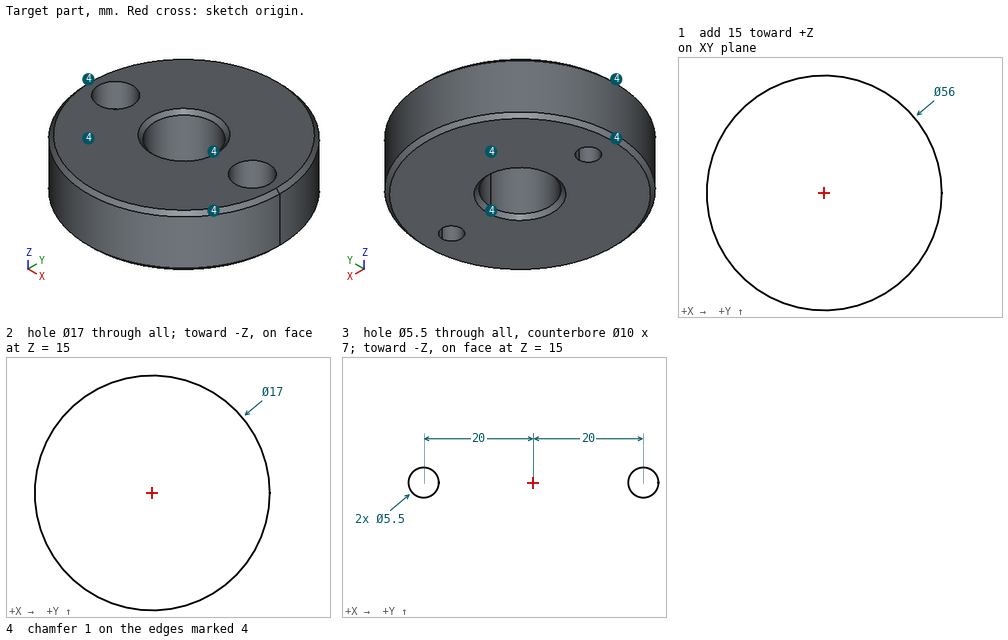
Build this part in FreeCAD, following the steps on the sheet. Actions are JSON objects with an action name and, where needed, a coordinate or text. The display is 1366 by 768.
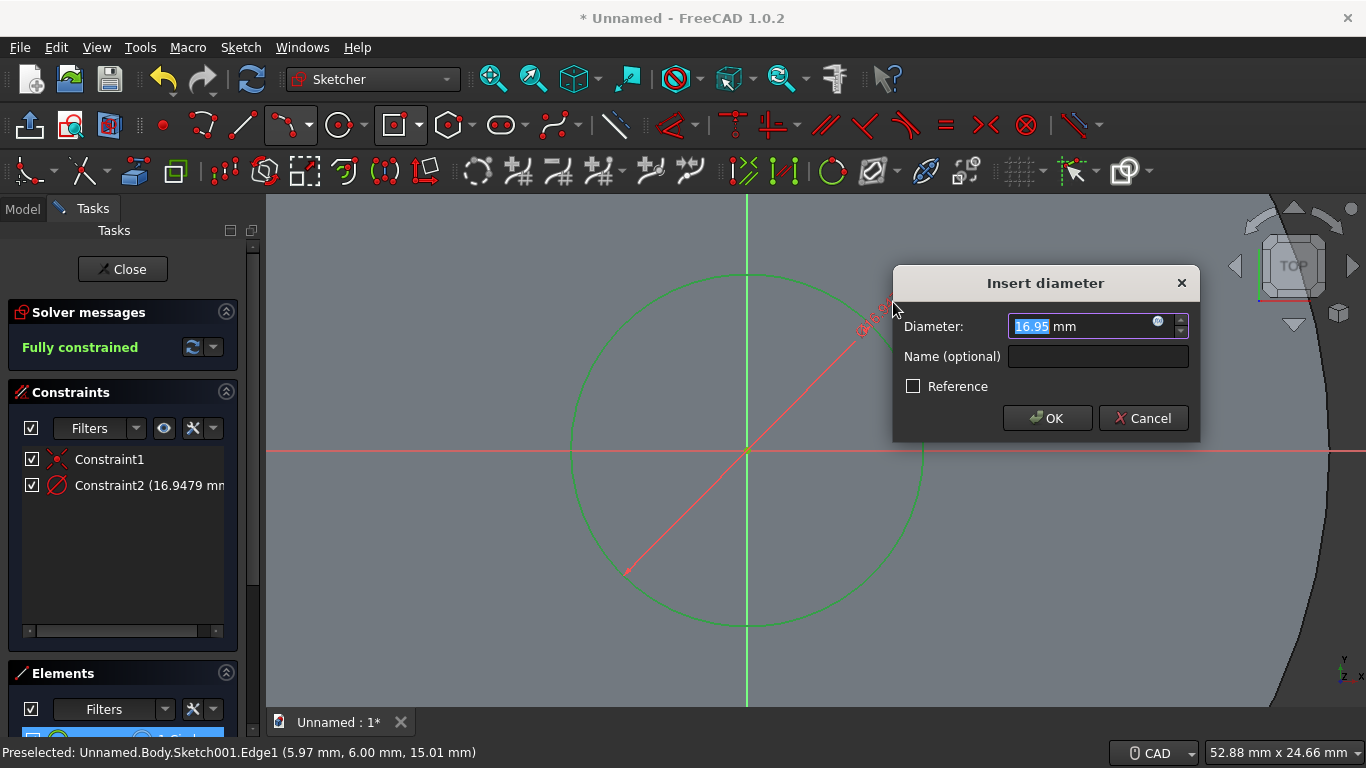
{"action": "type", "text": "17"}
{"action": "key", "text": "Return"}
{"action": "key", "text": "Escape"}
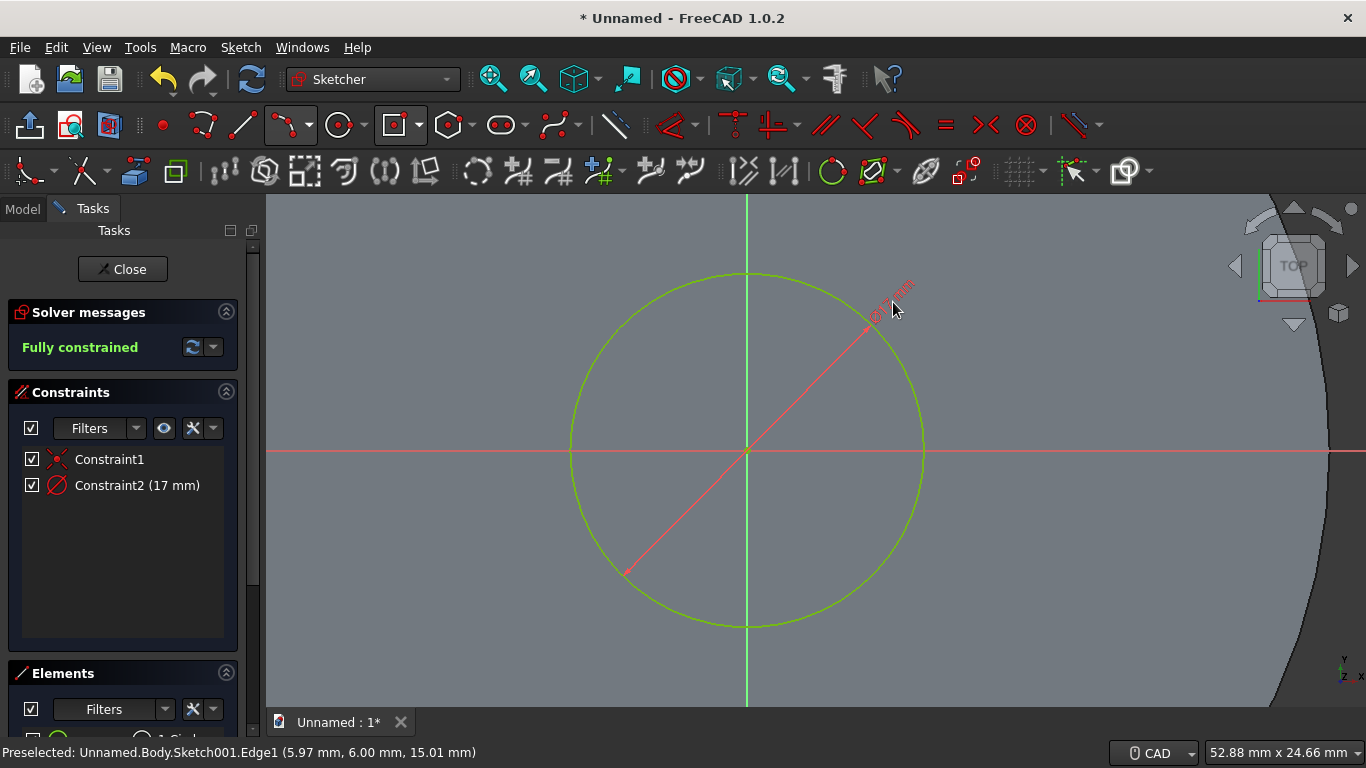
{"action": "left_click", "coordinate": [123, 269]}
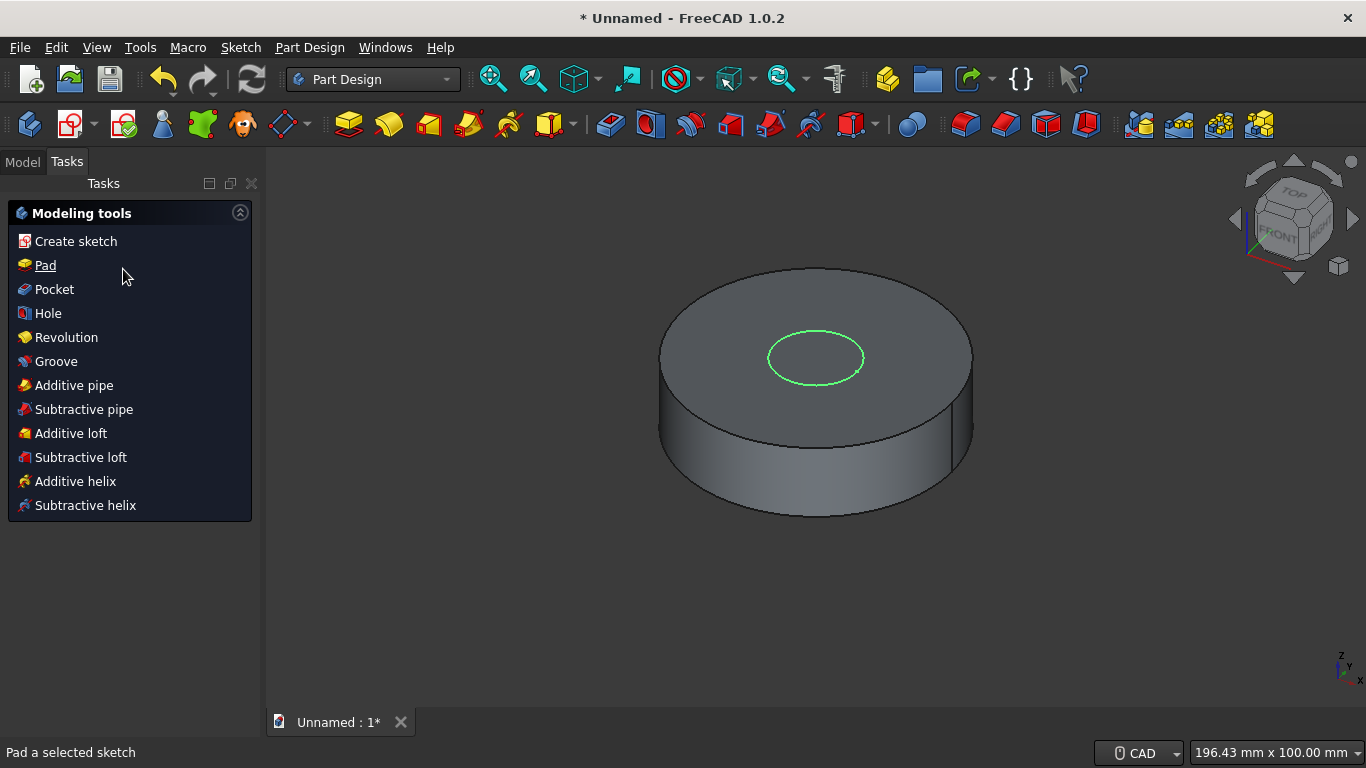
{"action": "left_click", "coordinate": [652, 124]}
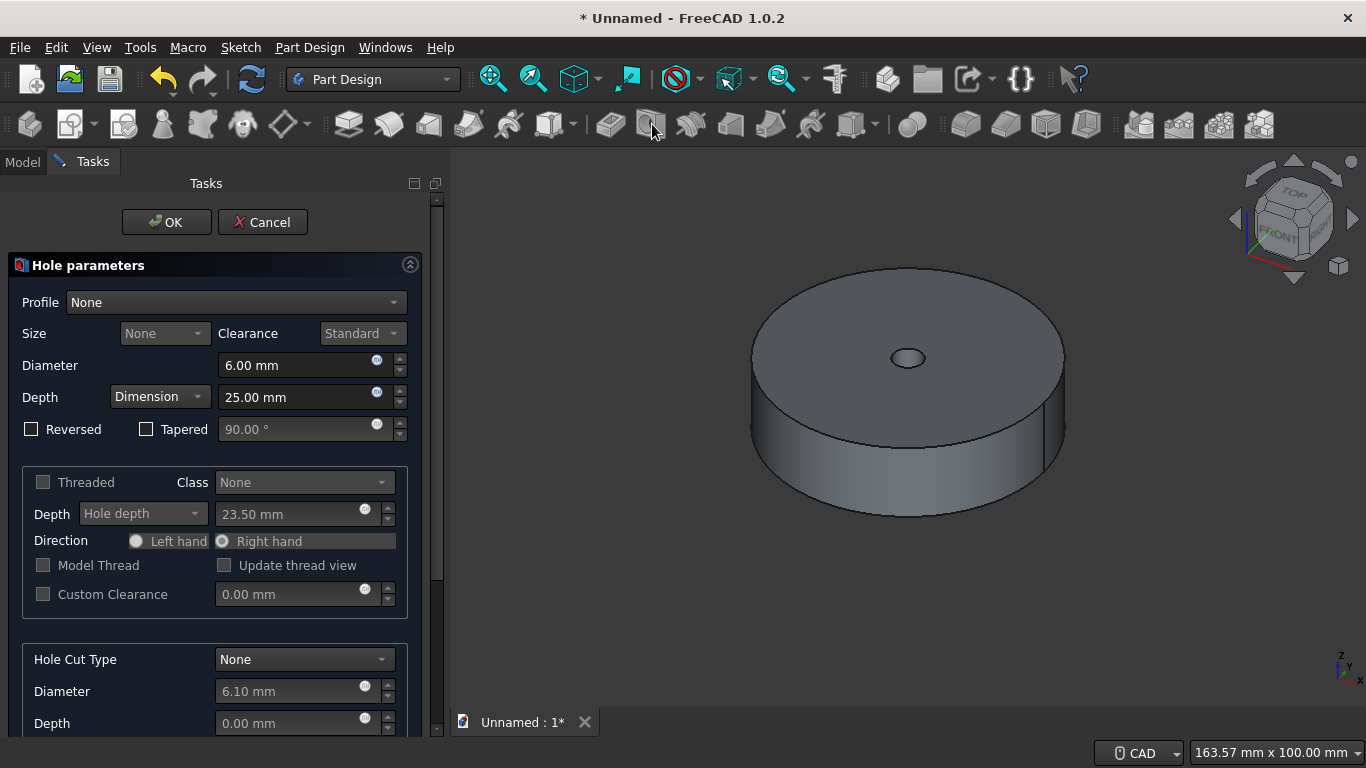
{"action": "triple_click", "coordinate": [305, 365]}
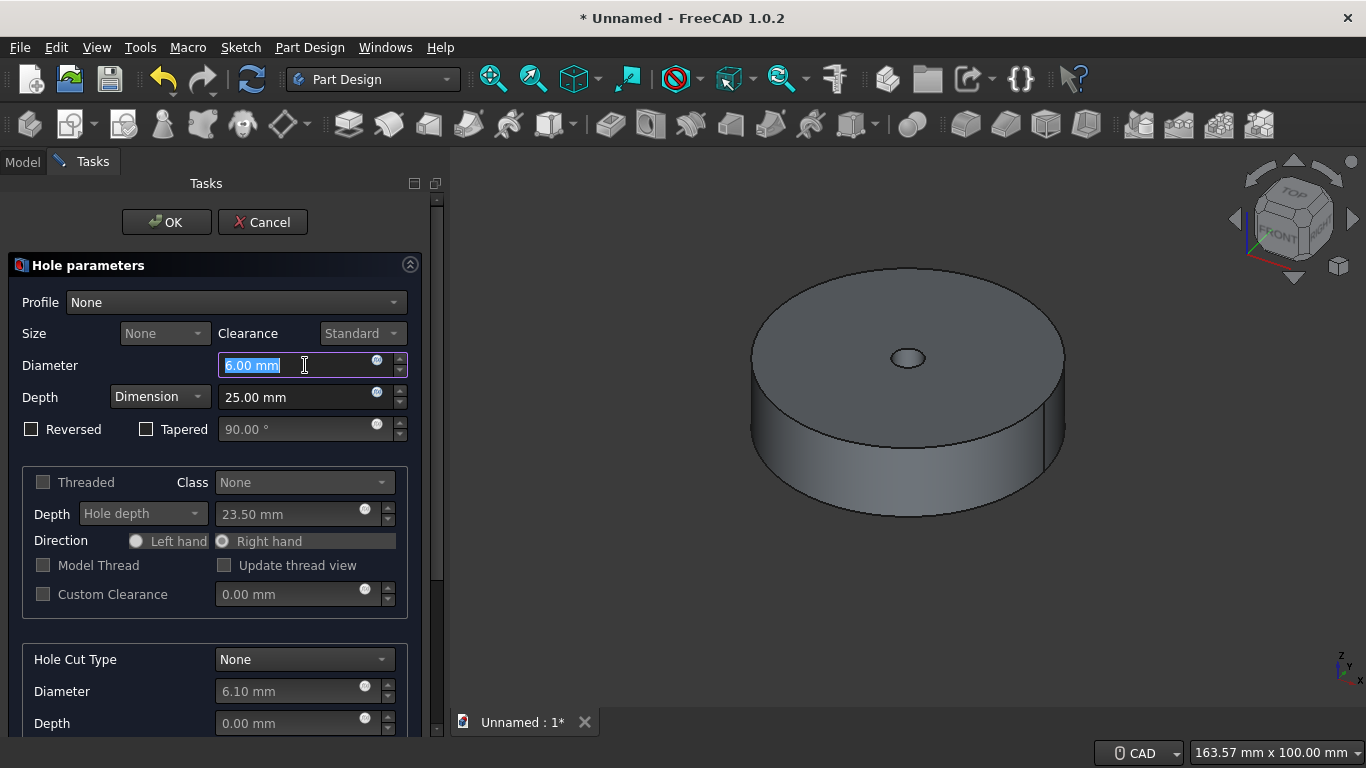
{"action": "type", "text": "17"}
{"action": "key", "text": "Tab"}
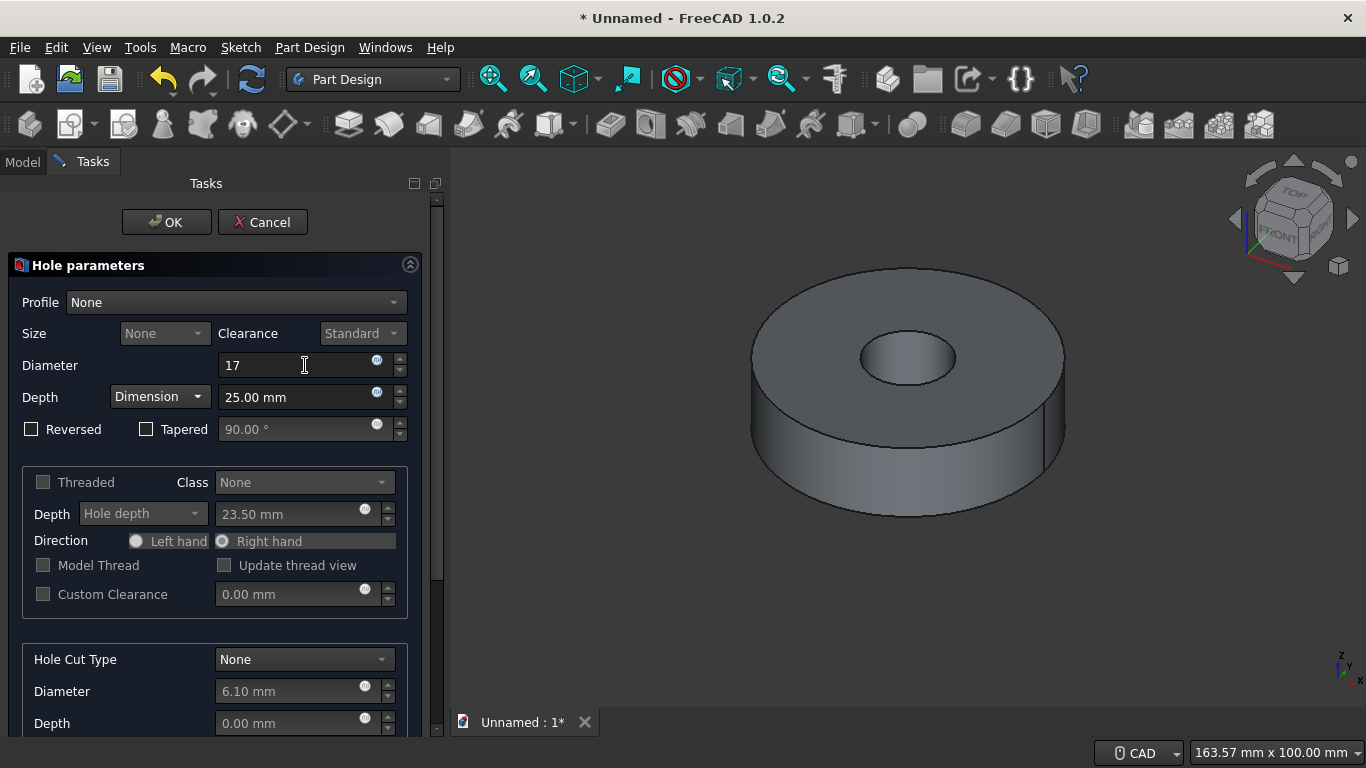
{"action": "left_click", "coordinate": [161, 396]}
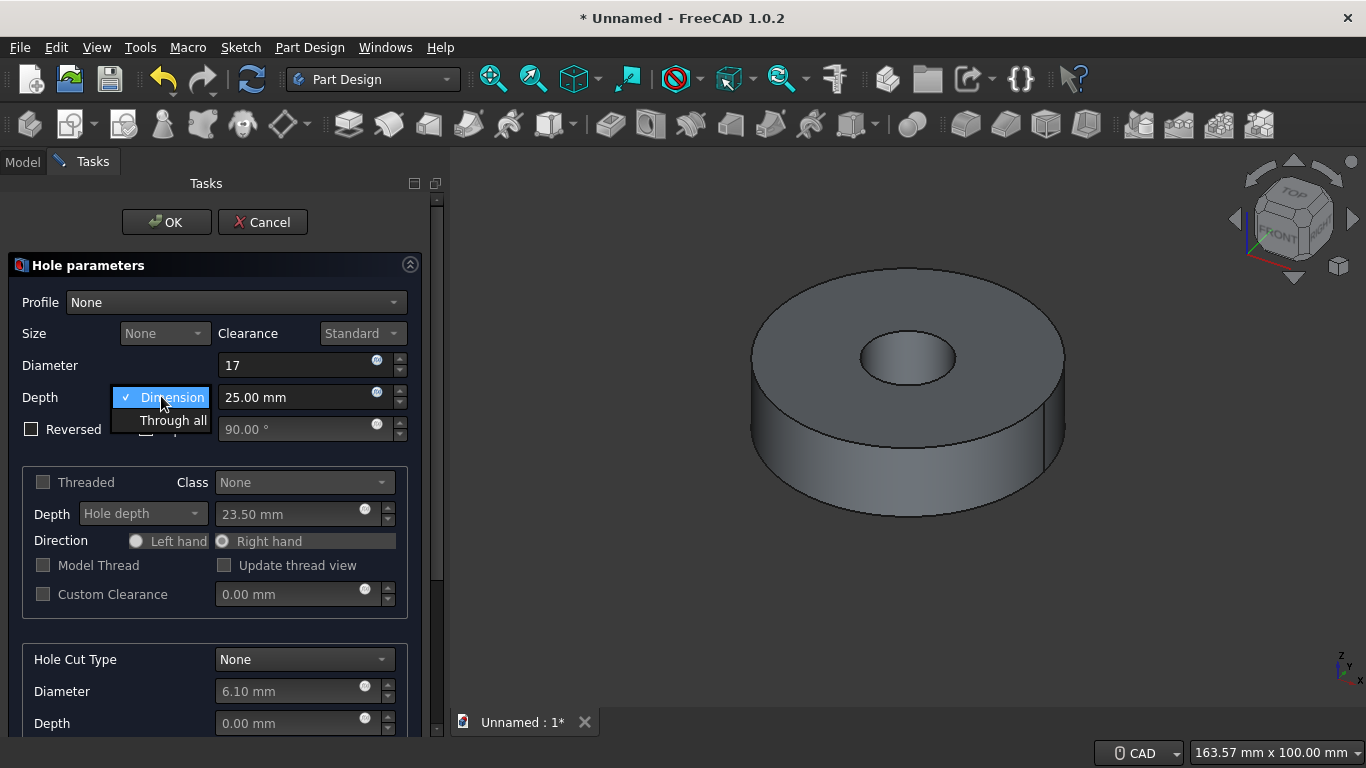
{"action": "left_click", "coordinate": [160, 420]}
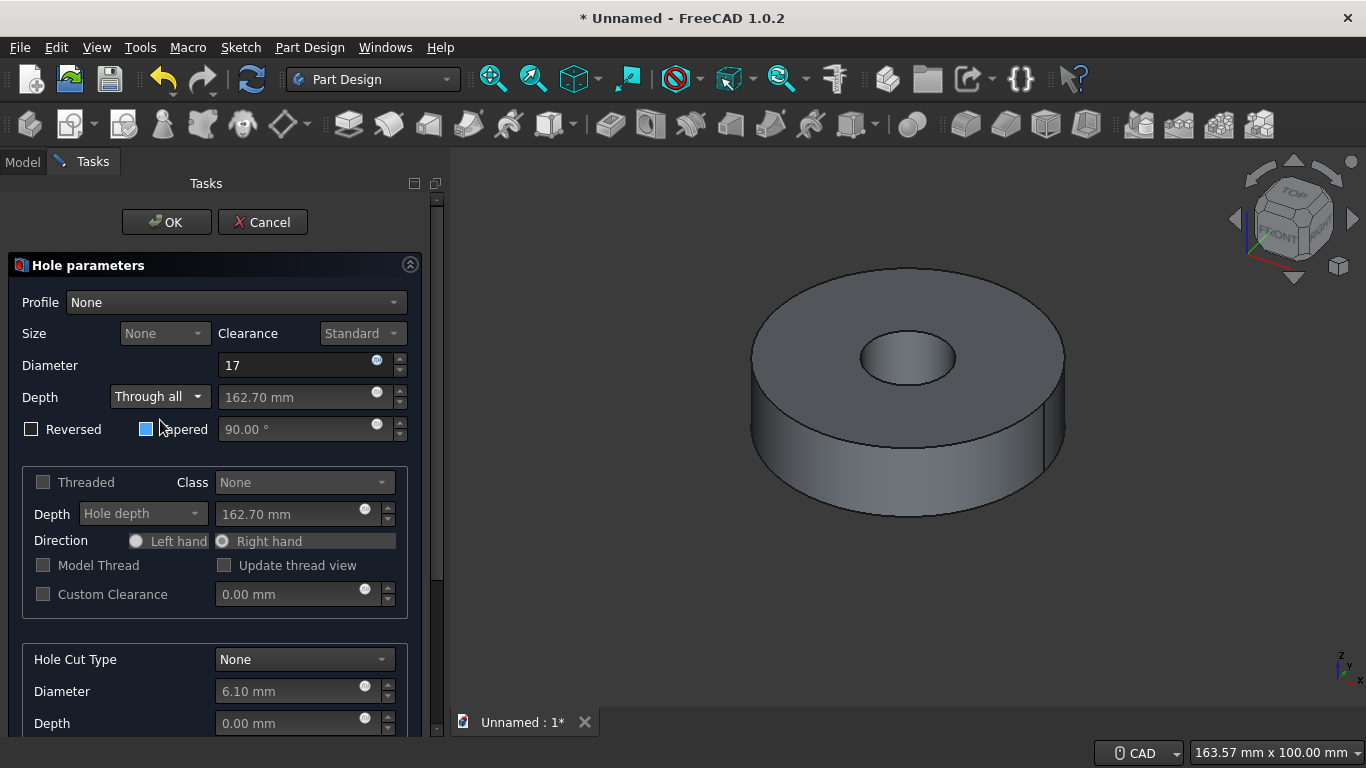
{"action": "left_click", "coordinate": [167, 222]}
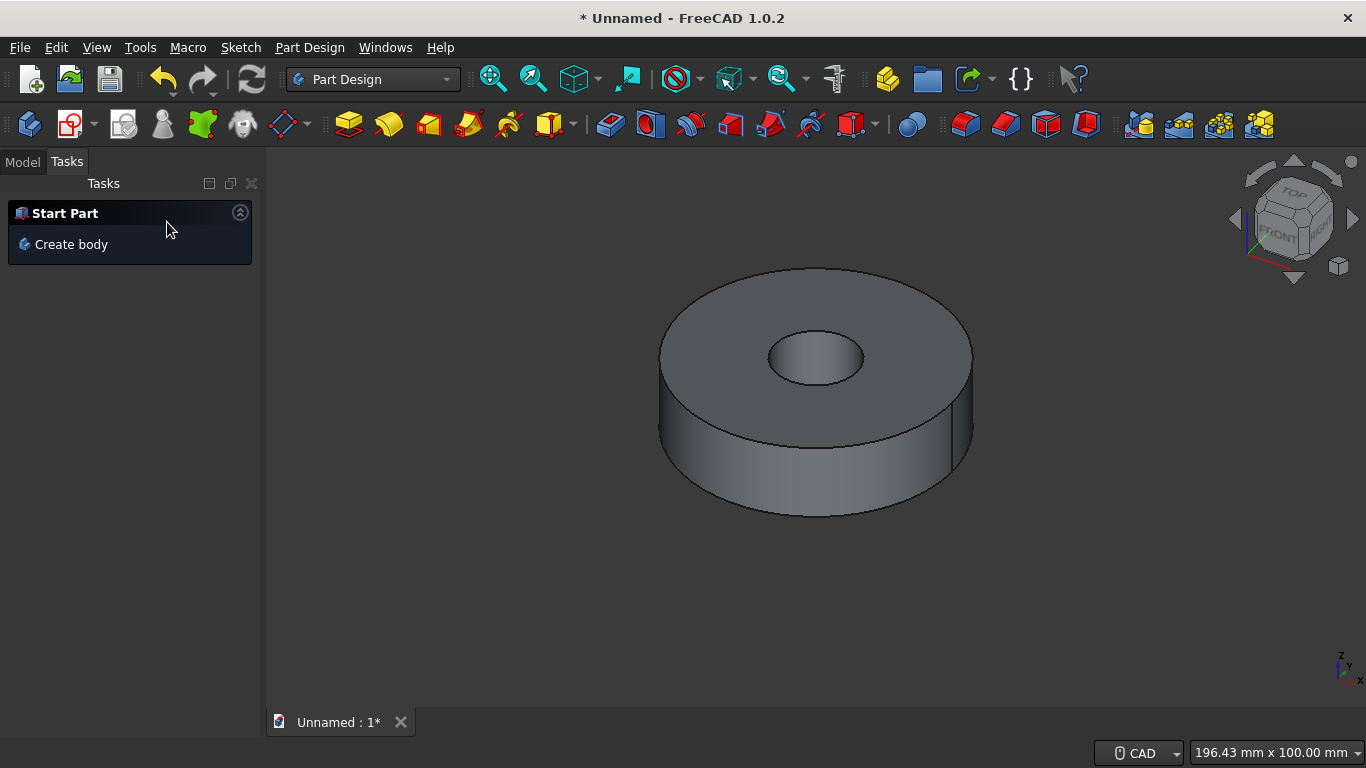
{"action": "left_click", "coordinate": [916, 361]}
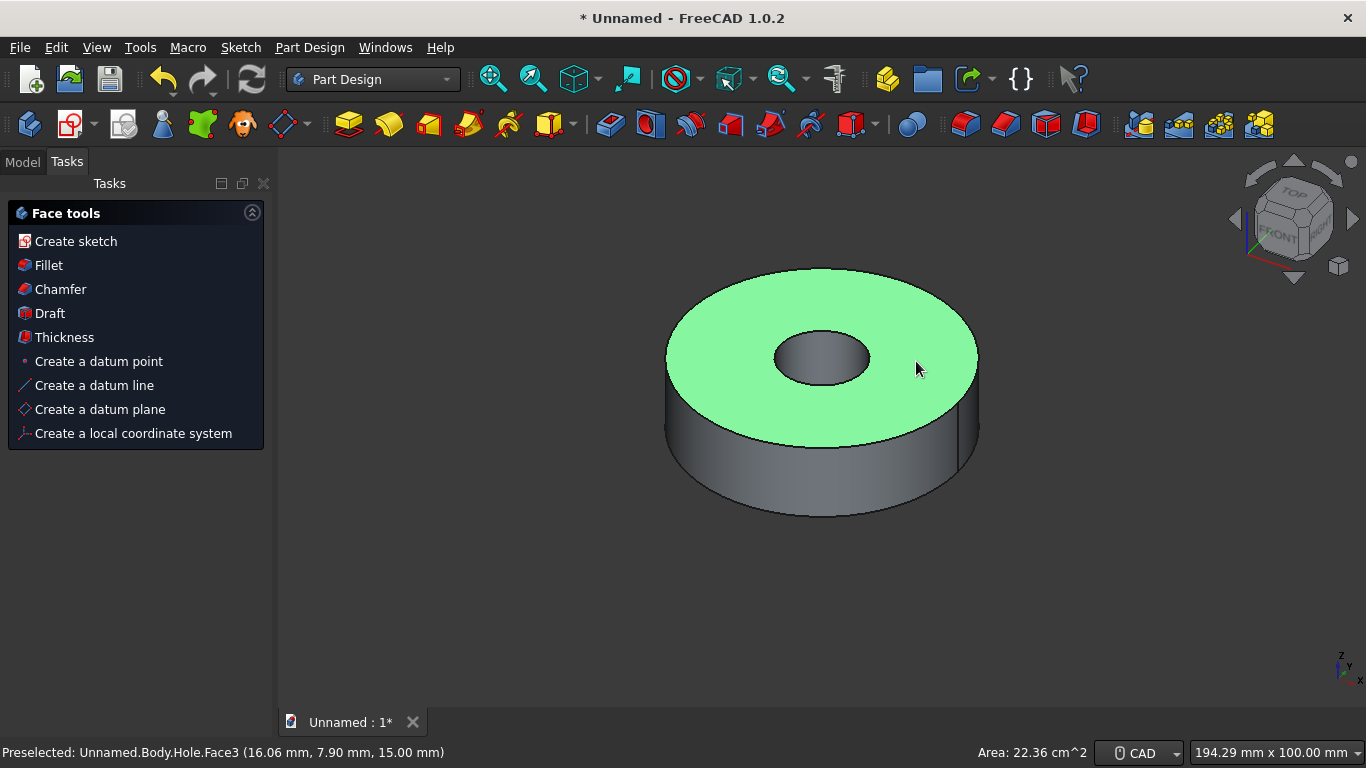
{"action": "left_click", "coordinate": [70, 124]}